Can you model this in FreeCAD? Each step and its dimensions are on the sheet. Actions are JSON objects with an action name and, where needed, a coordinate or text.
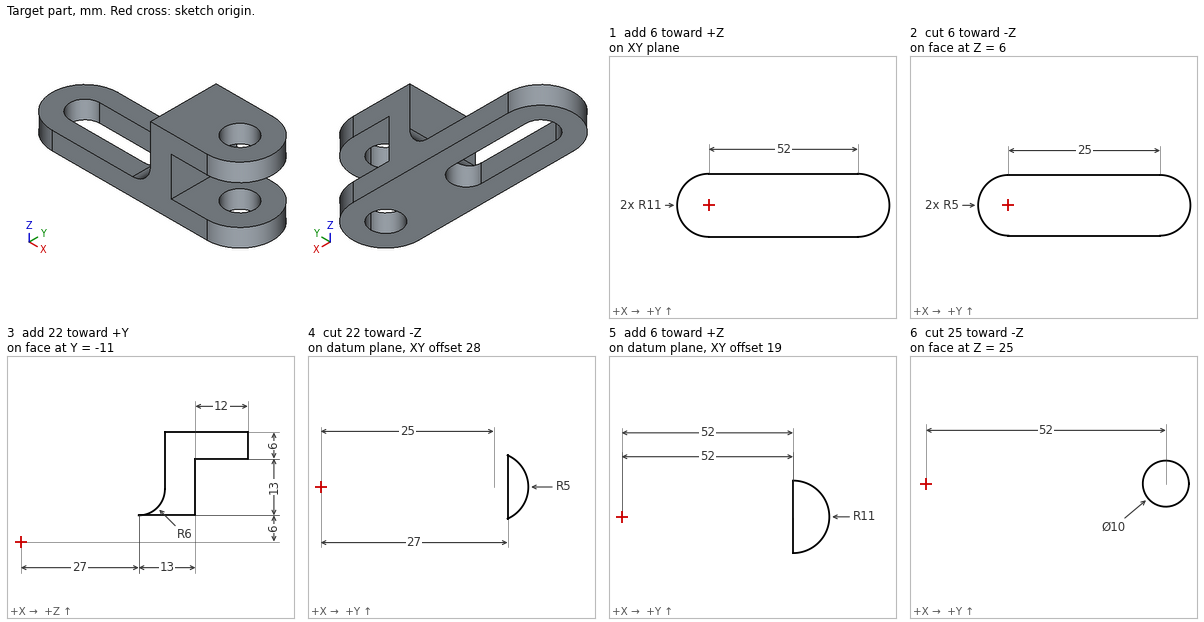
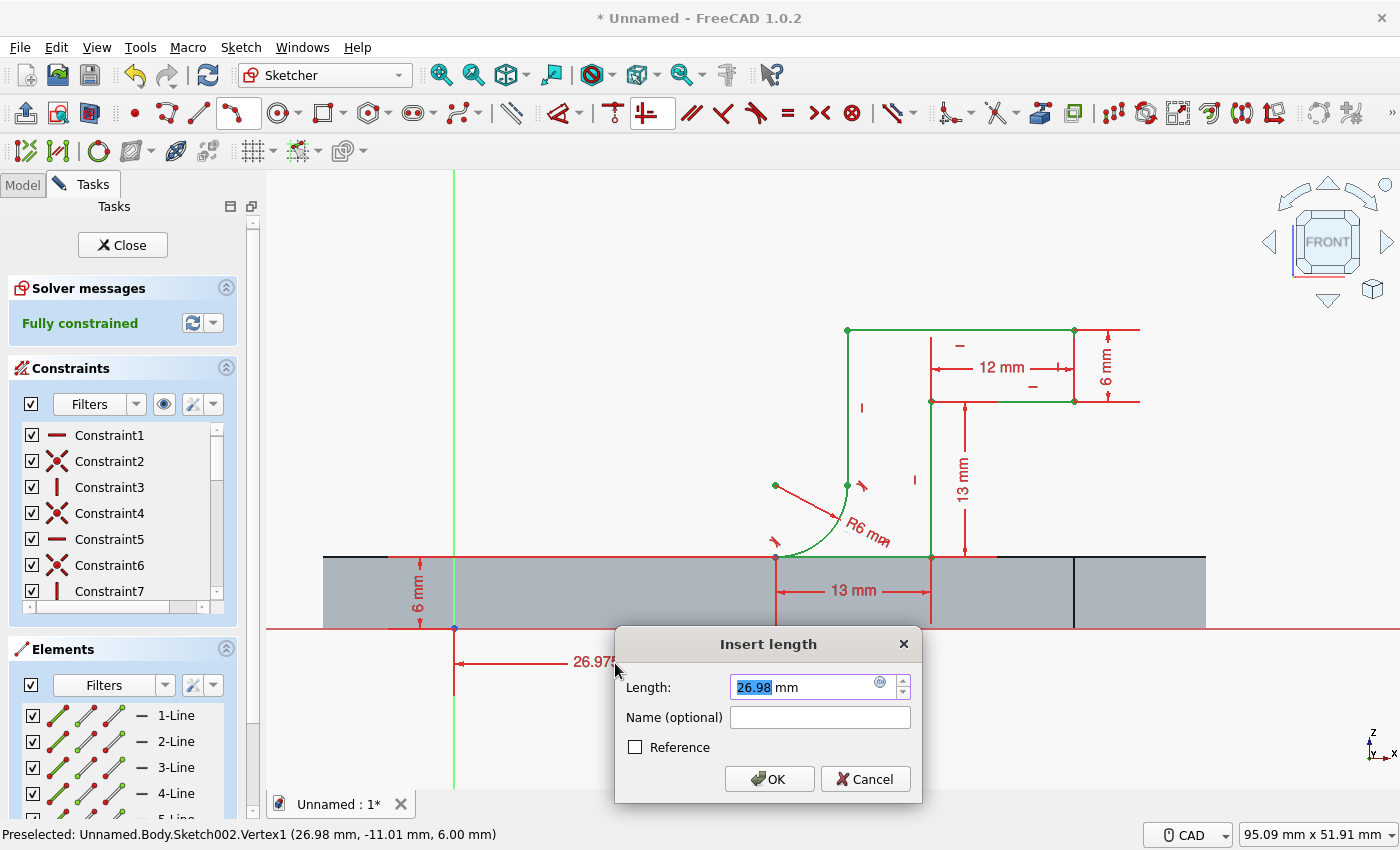
{"action": "type", "text": "27"}
{"action": "key", "text": "Return"}
{"action": "key", "text": "Escape"}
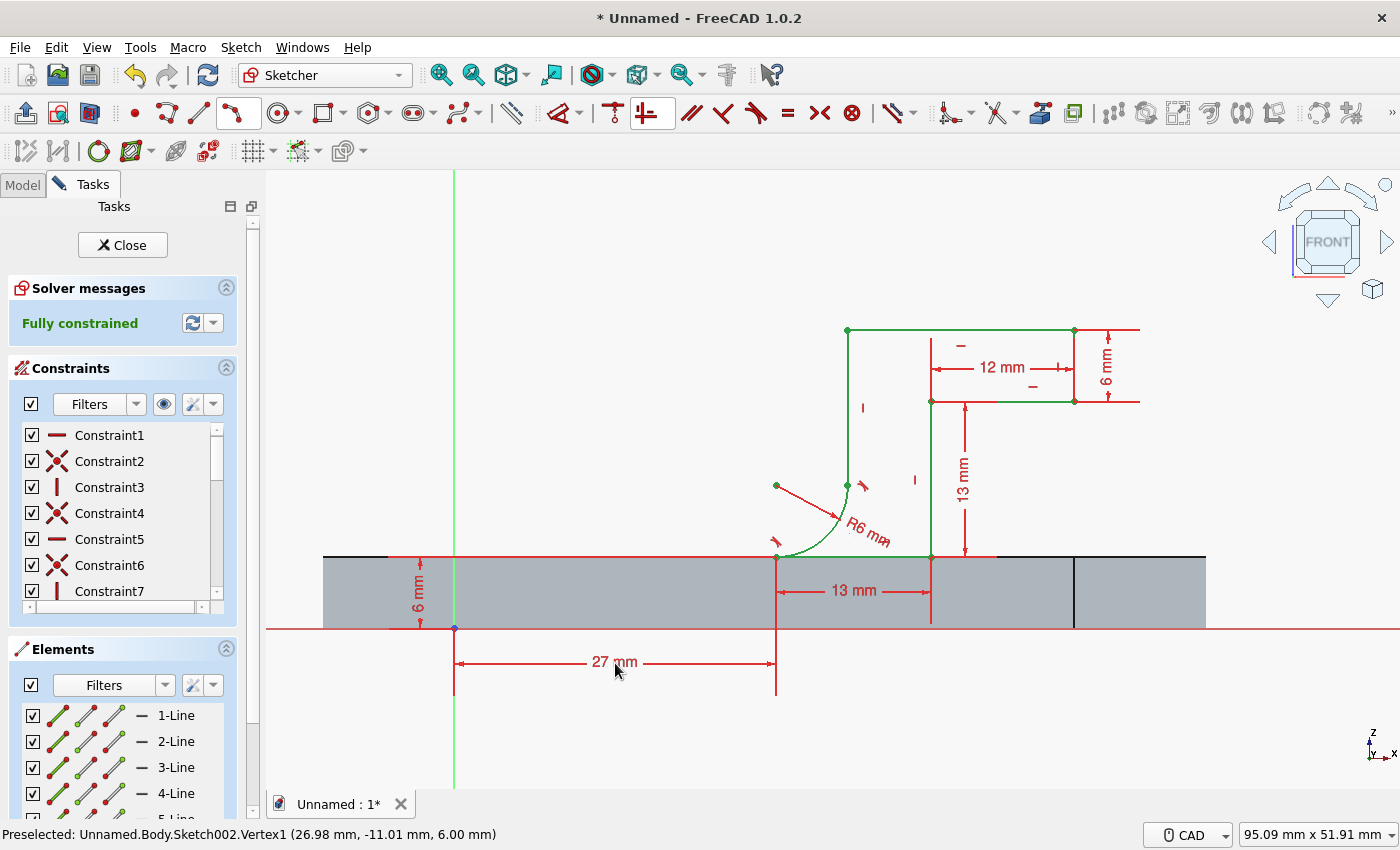
{"action": "left_click", "coordinate": [123, 245]}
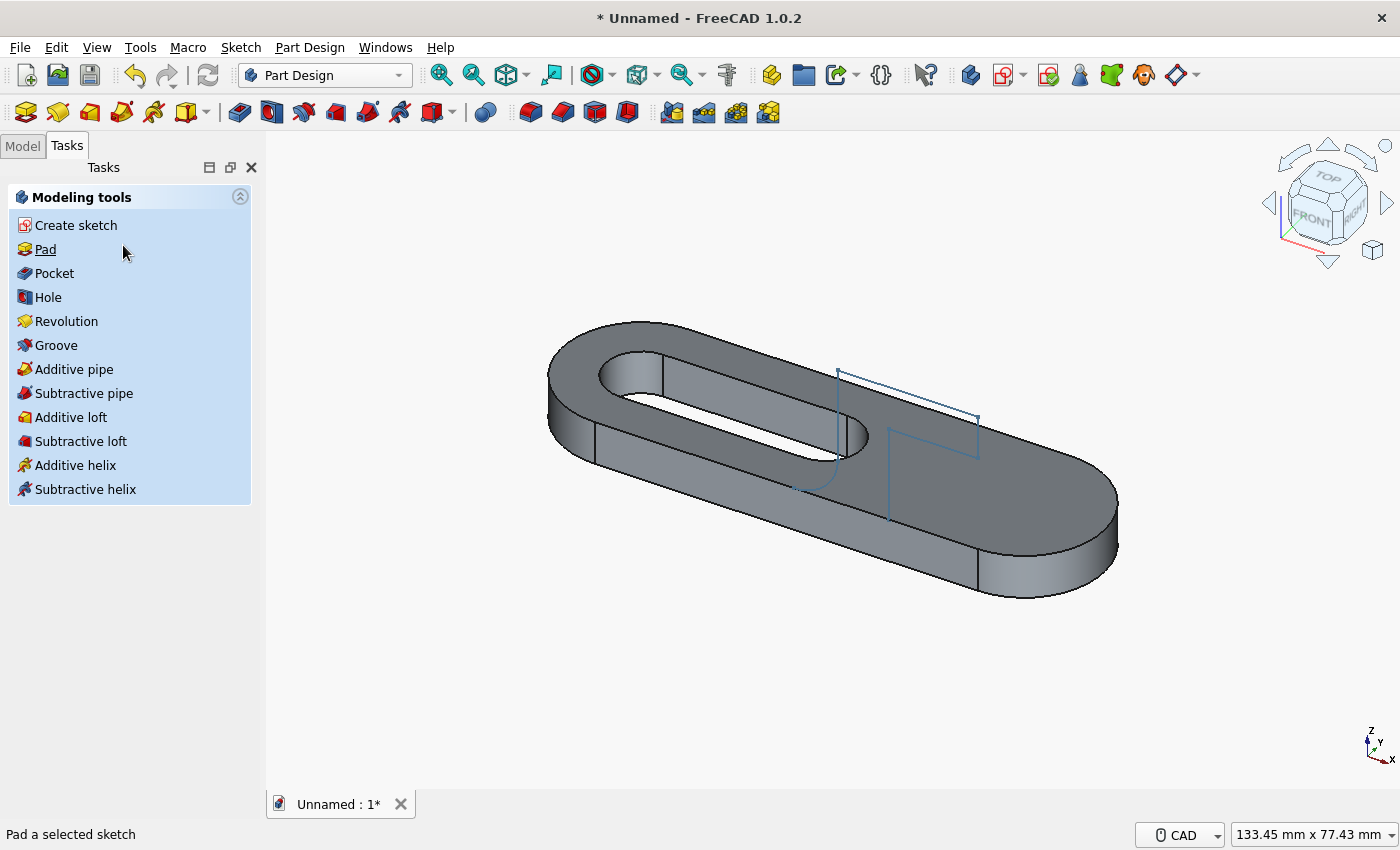
{"action": "left_click", "coordinate": [26, 112]}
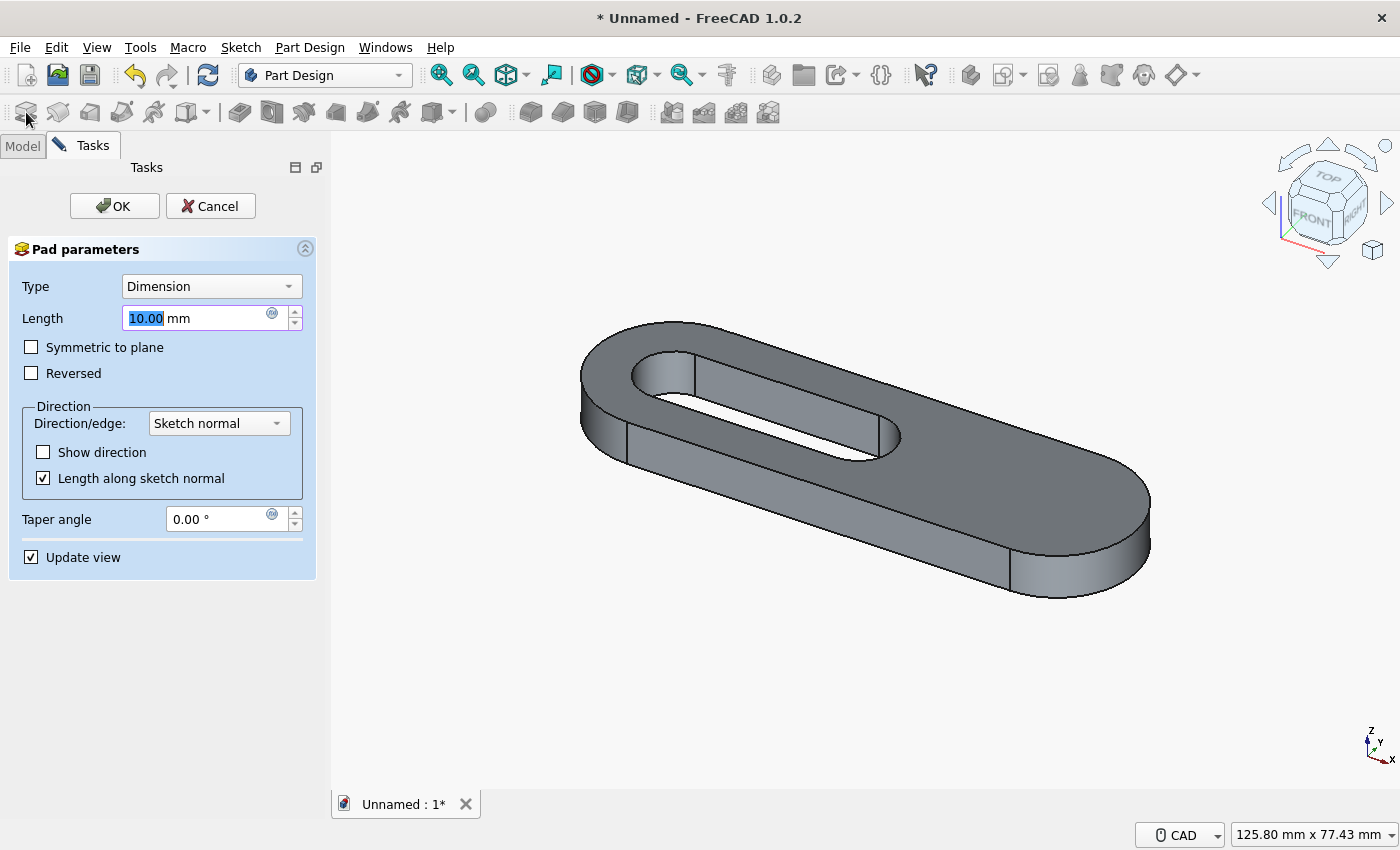
{"action": "type", "text": "22"}
{"action": "key", "text": "Tab"}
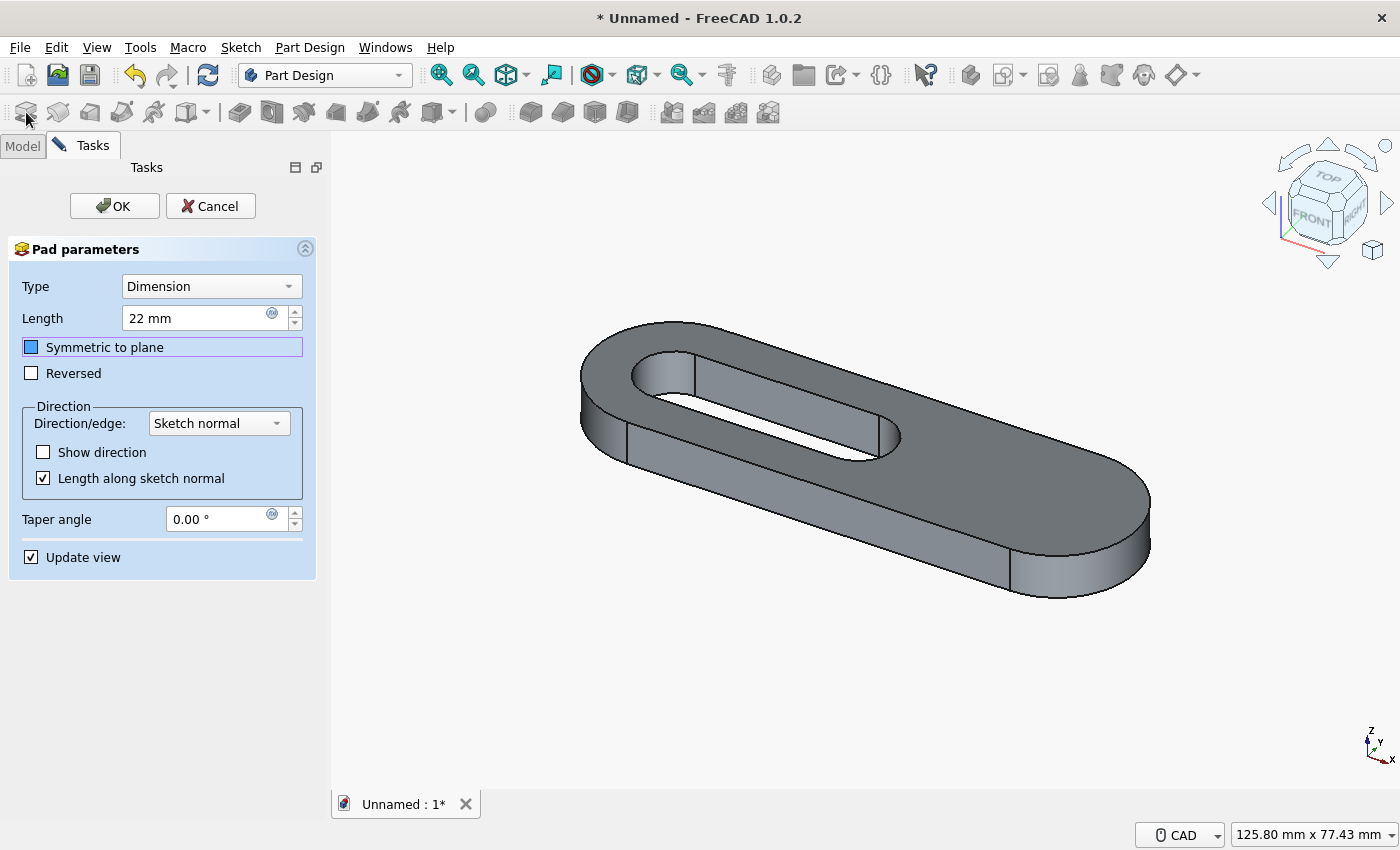
{"action": "left_click", "coordinate": [30, 373]}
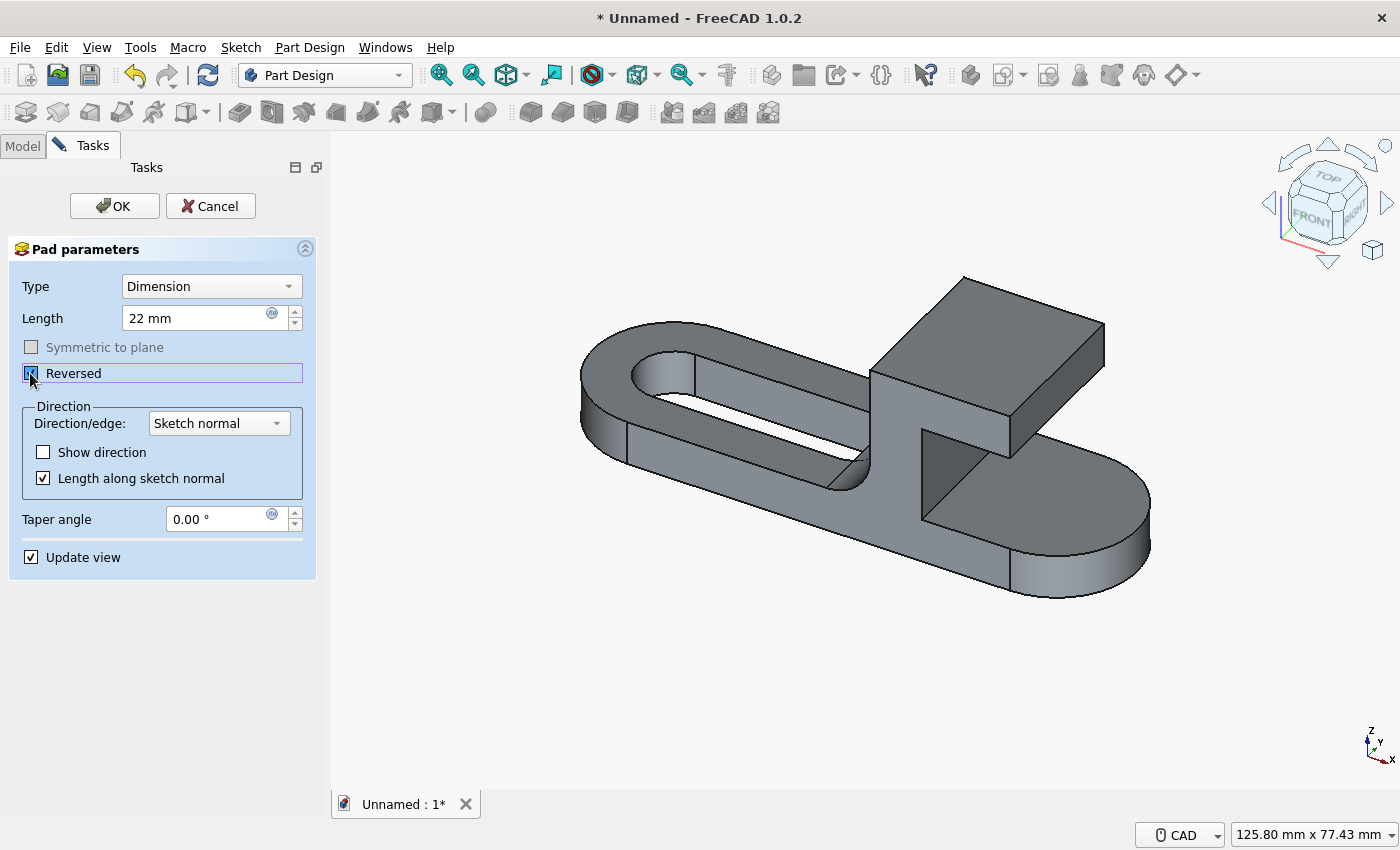
{"action": "left_click", "coordinate": [115, 206]}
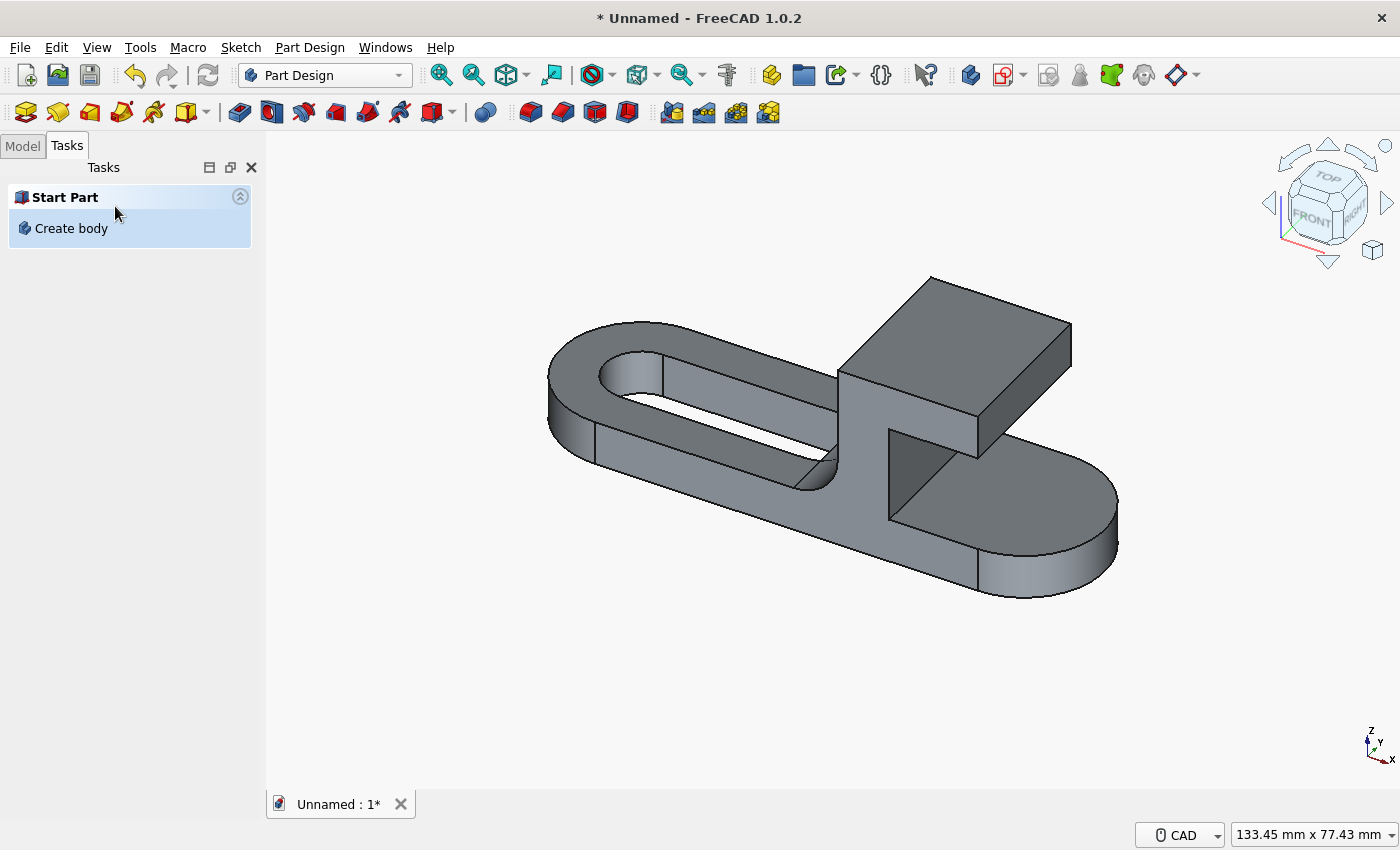
{"action": "left_click", "coordinate": [23, 145]}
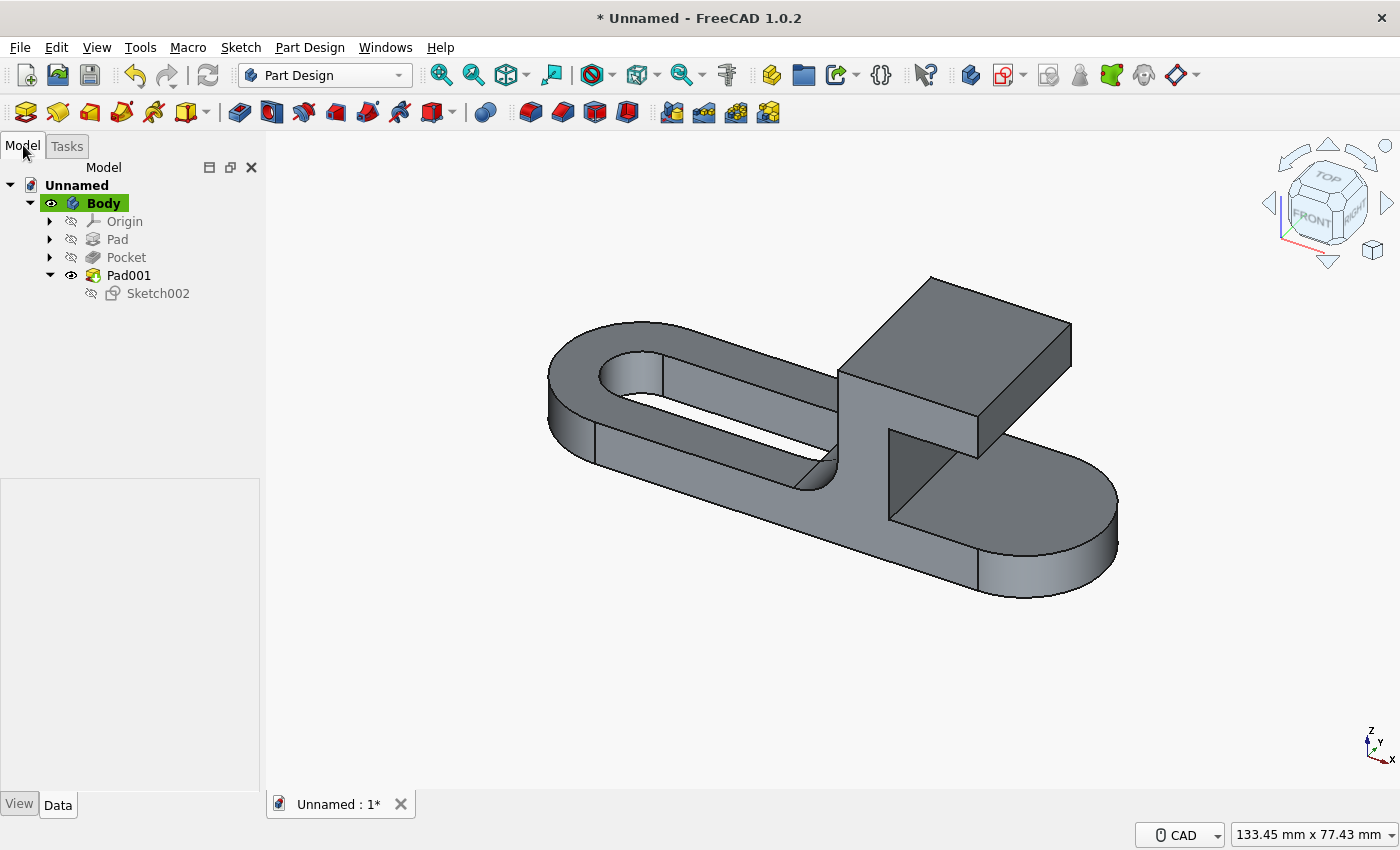
{"action": "left_click", "coordinate": [50, 221]}